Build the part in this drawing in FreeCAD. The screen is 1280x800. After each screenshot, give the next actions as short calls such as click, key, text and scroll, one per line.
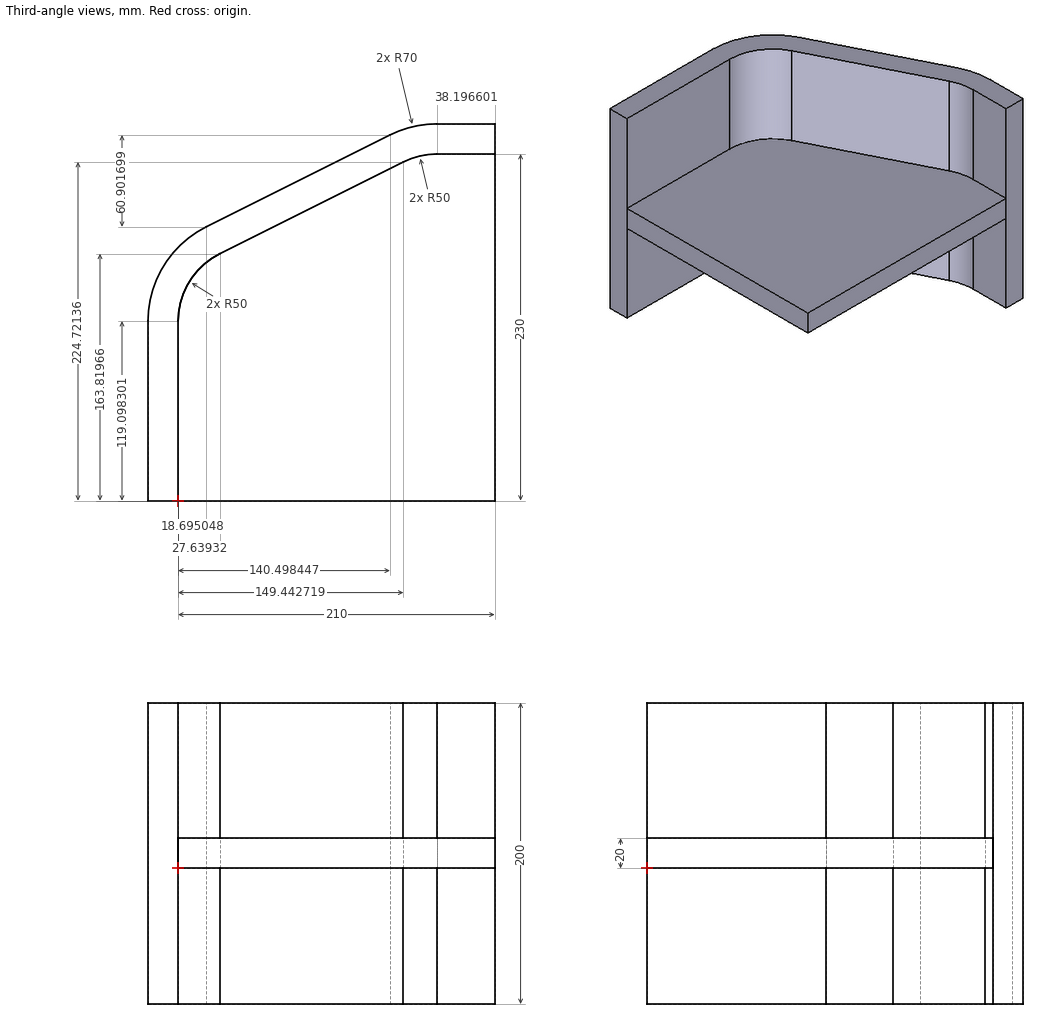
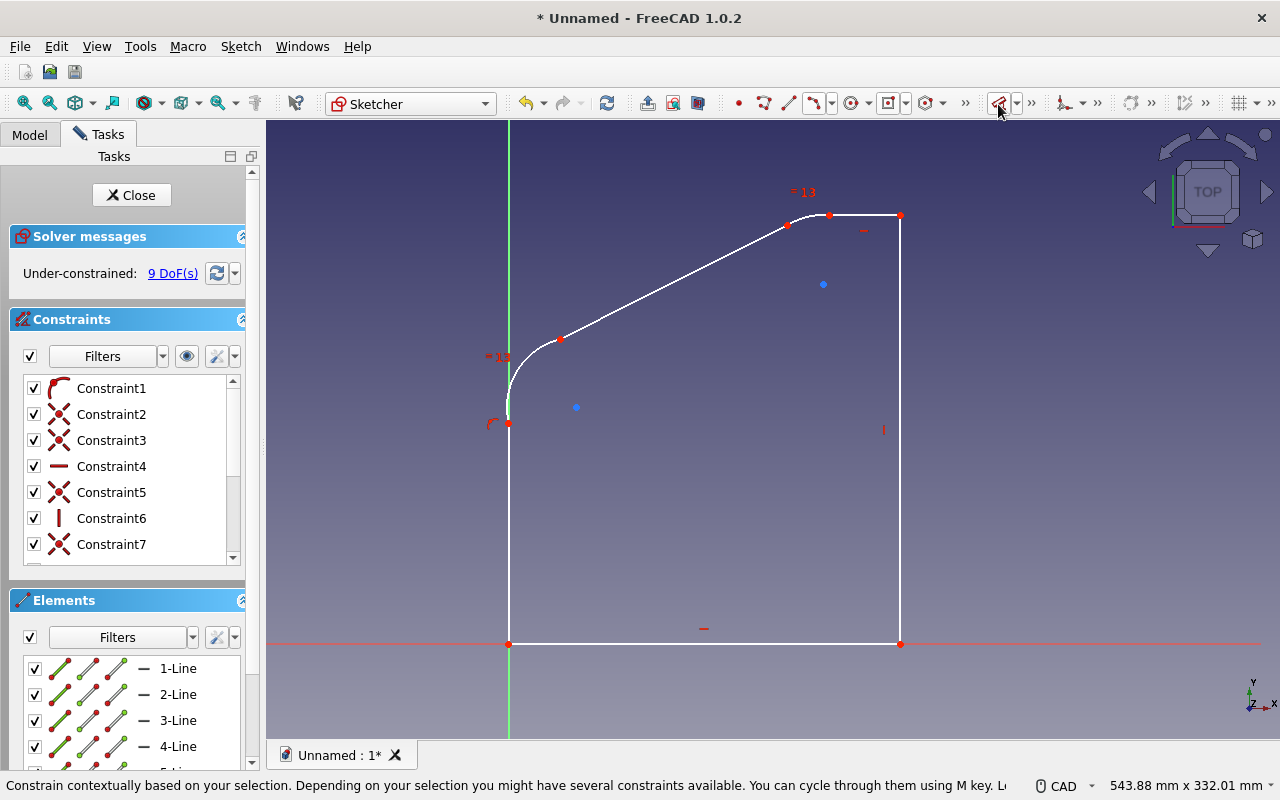
click(531, 354)
click(555, 307)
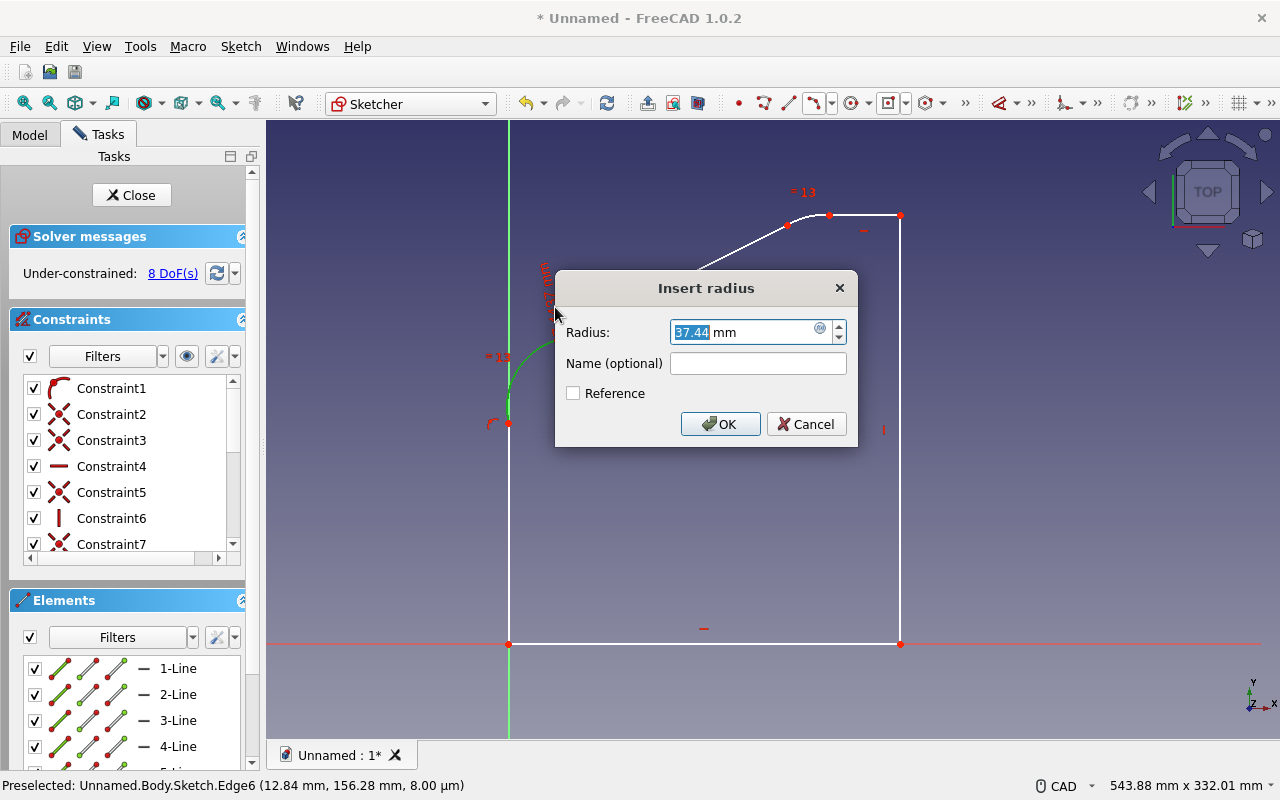
text(50)
key(Return)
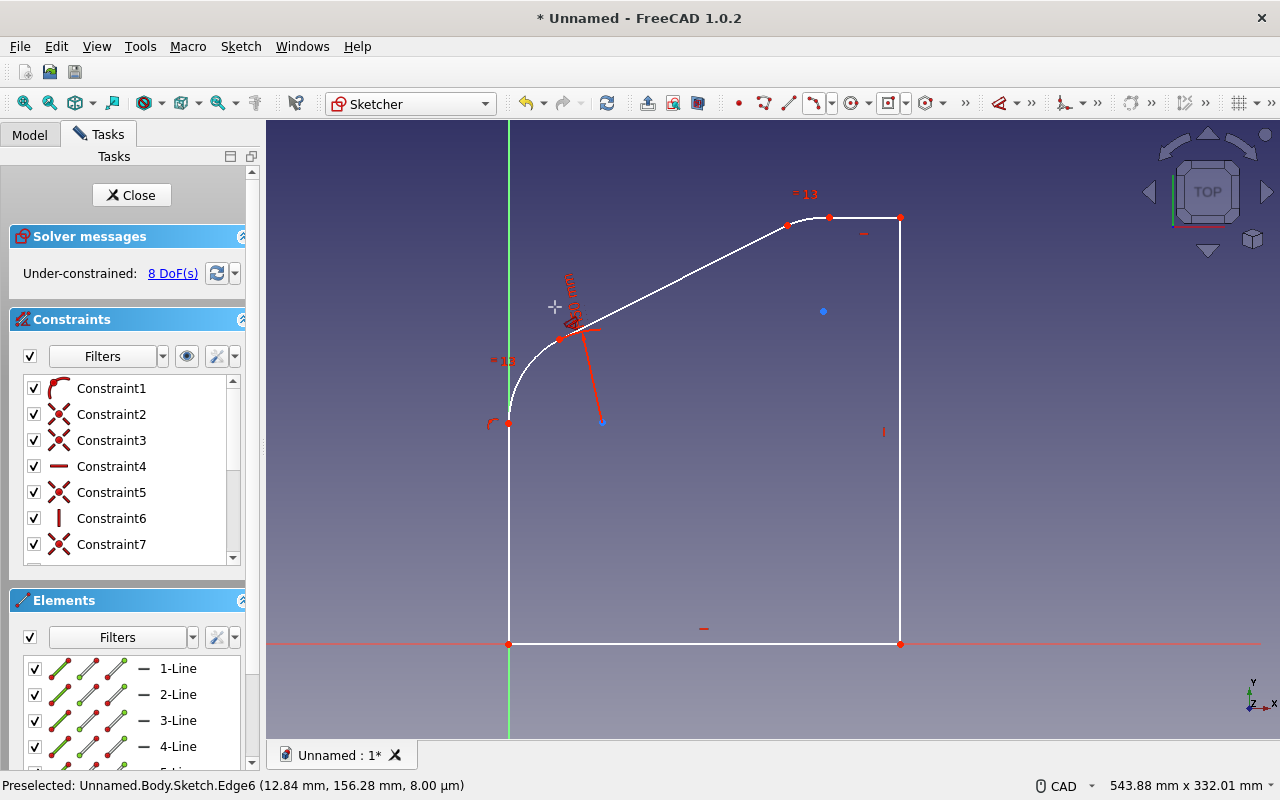
click(626, 644)
click(704, 678)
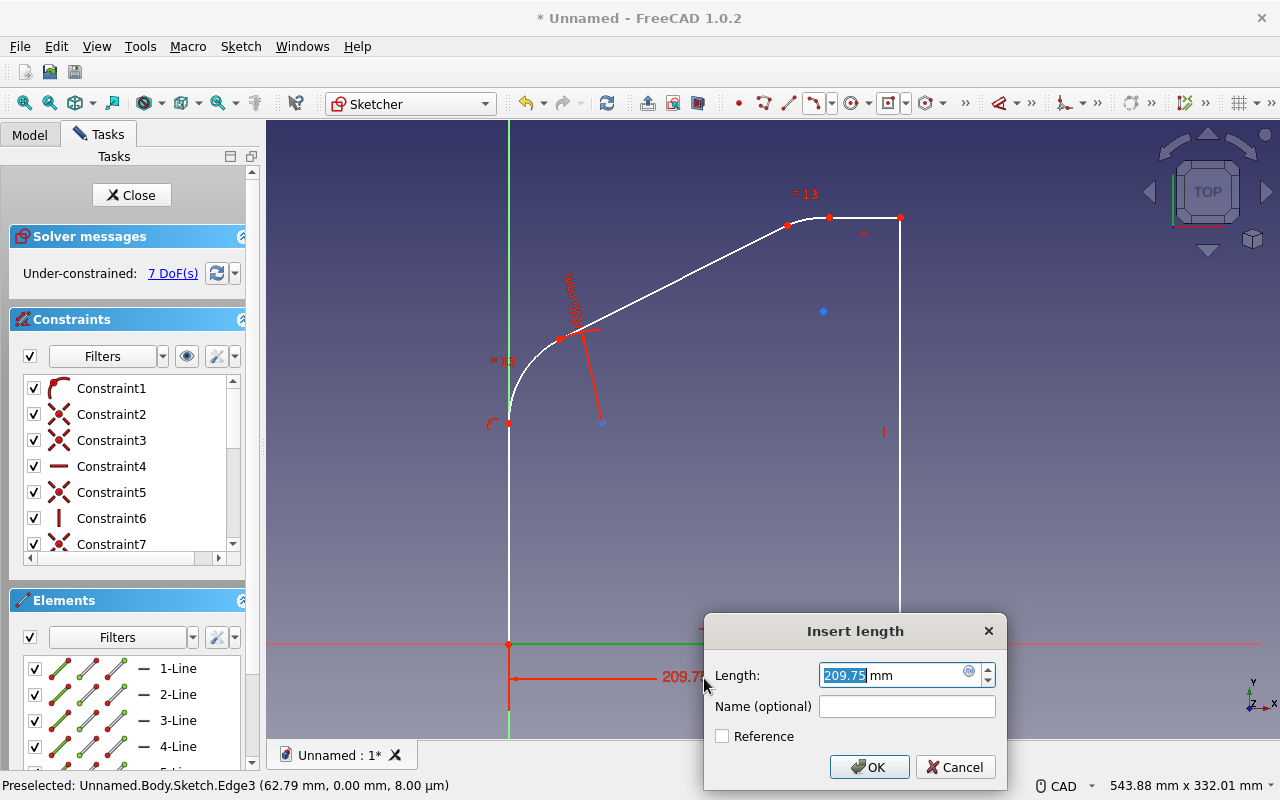
text(210)
key(Return)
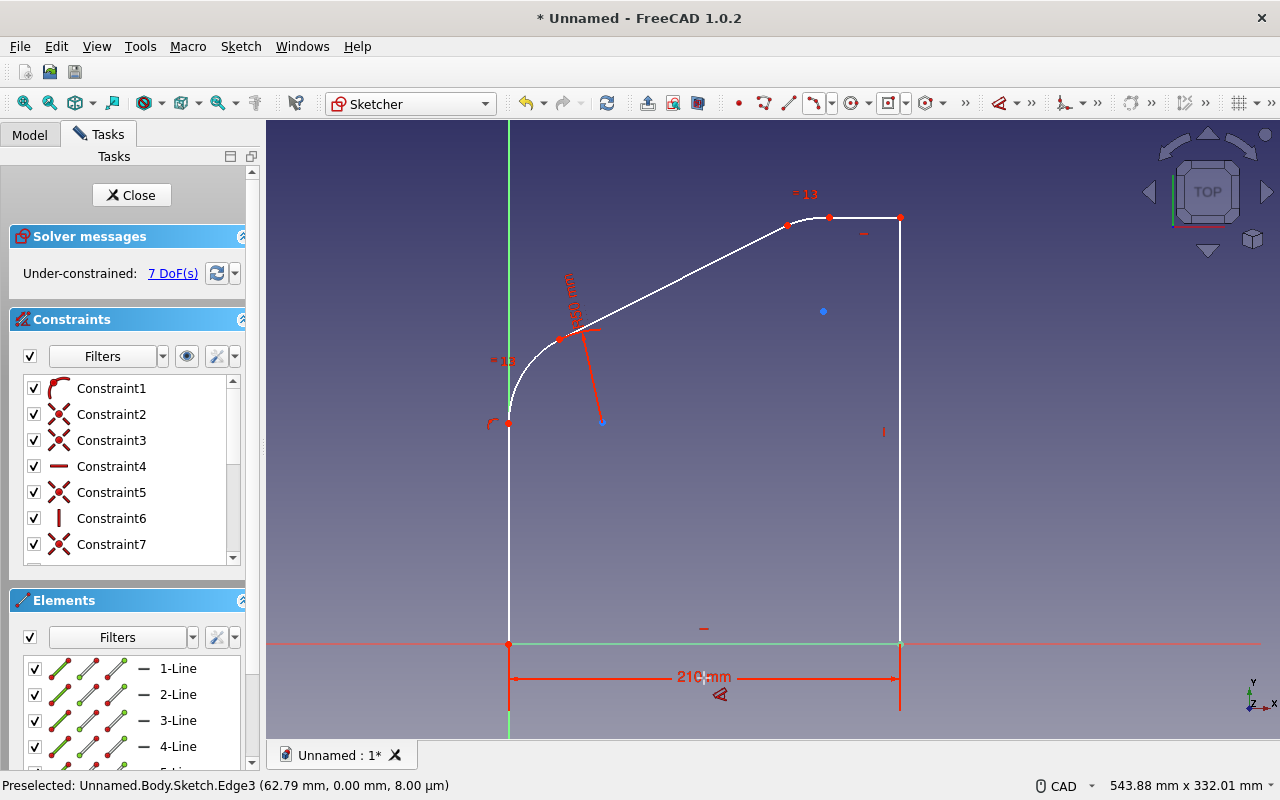
click(900, 516)
click(934, 431)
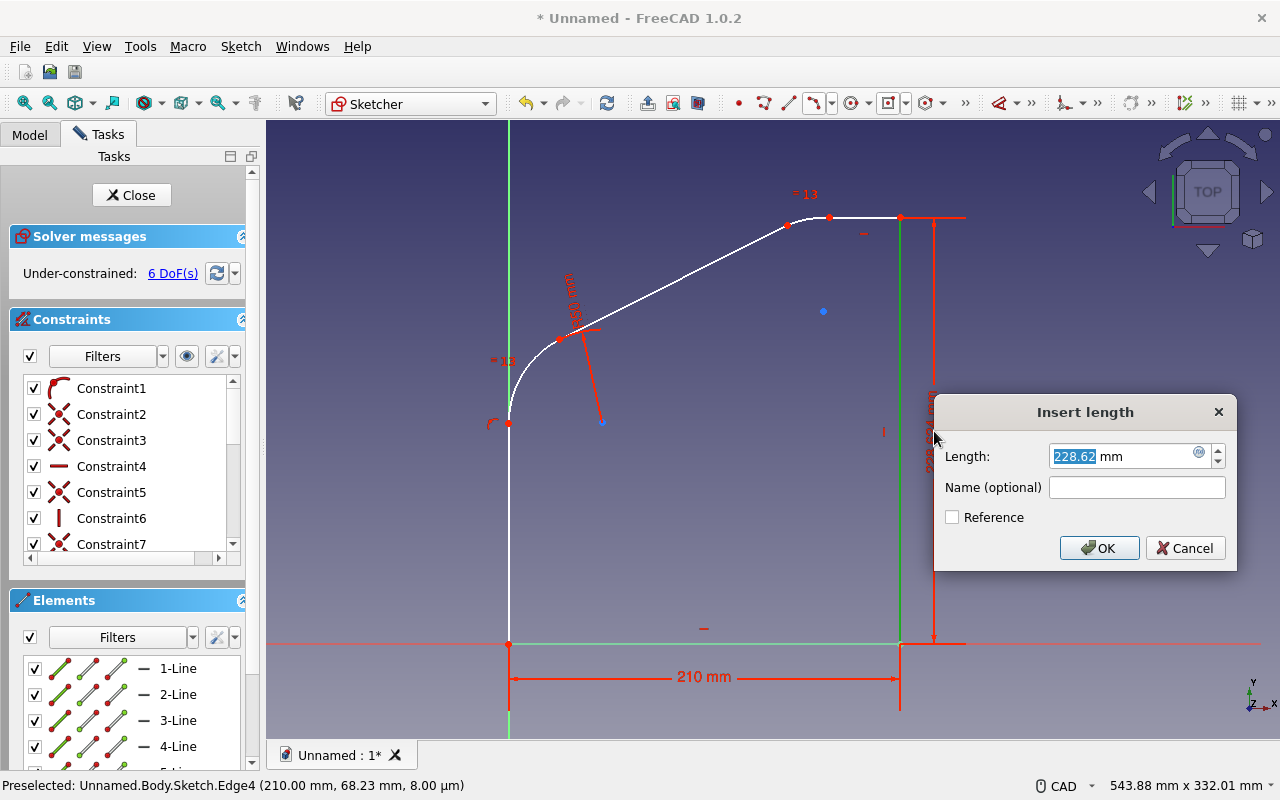
text(230)
key(Return)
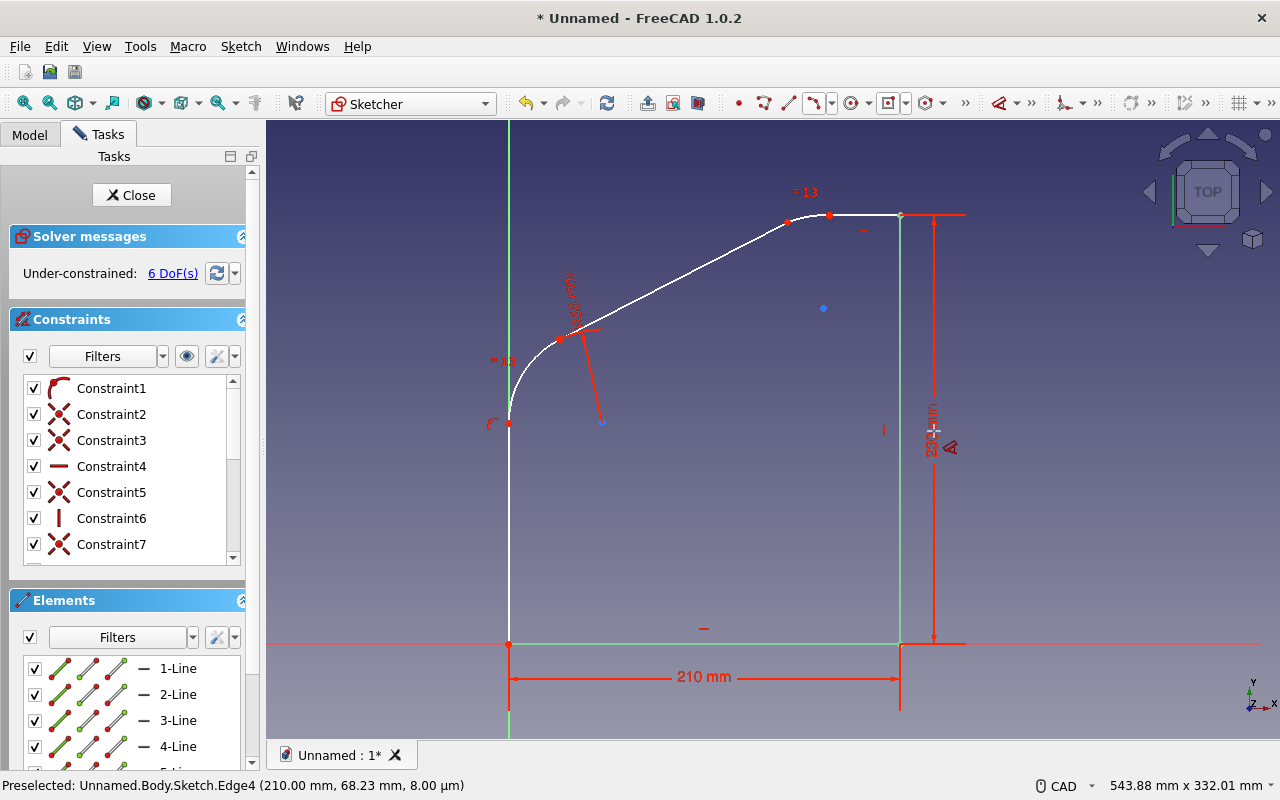
click(879, 215)
click(865, 181)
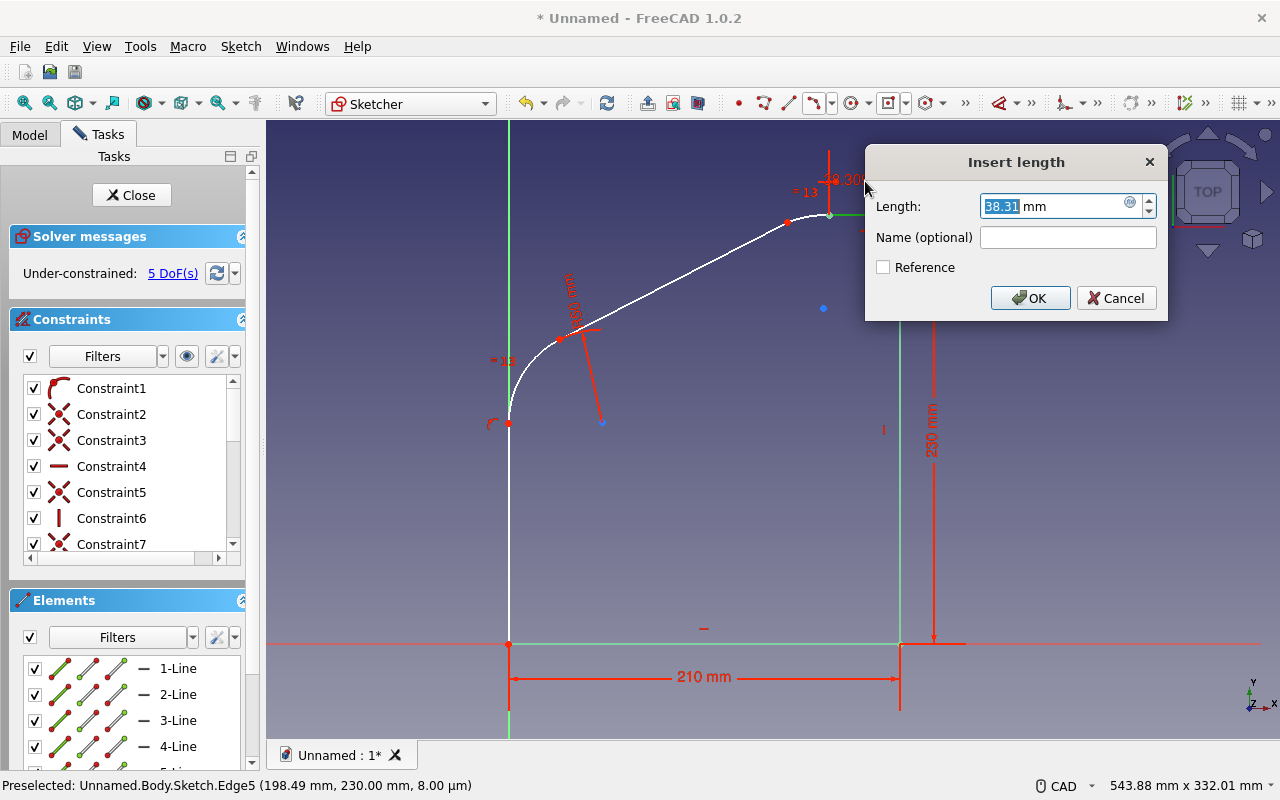
text(38.196601)
key(Return)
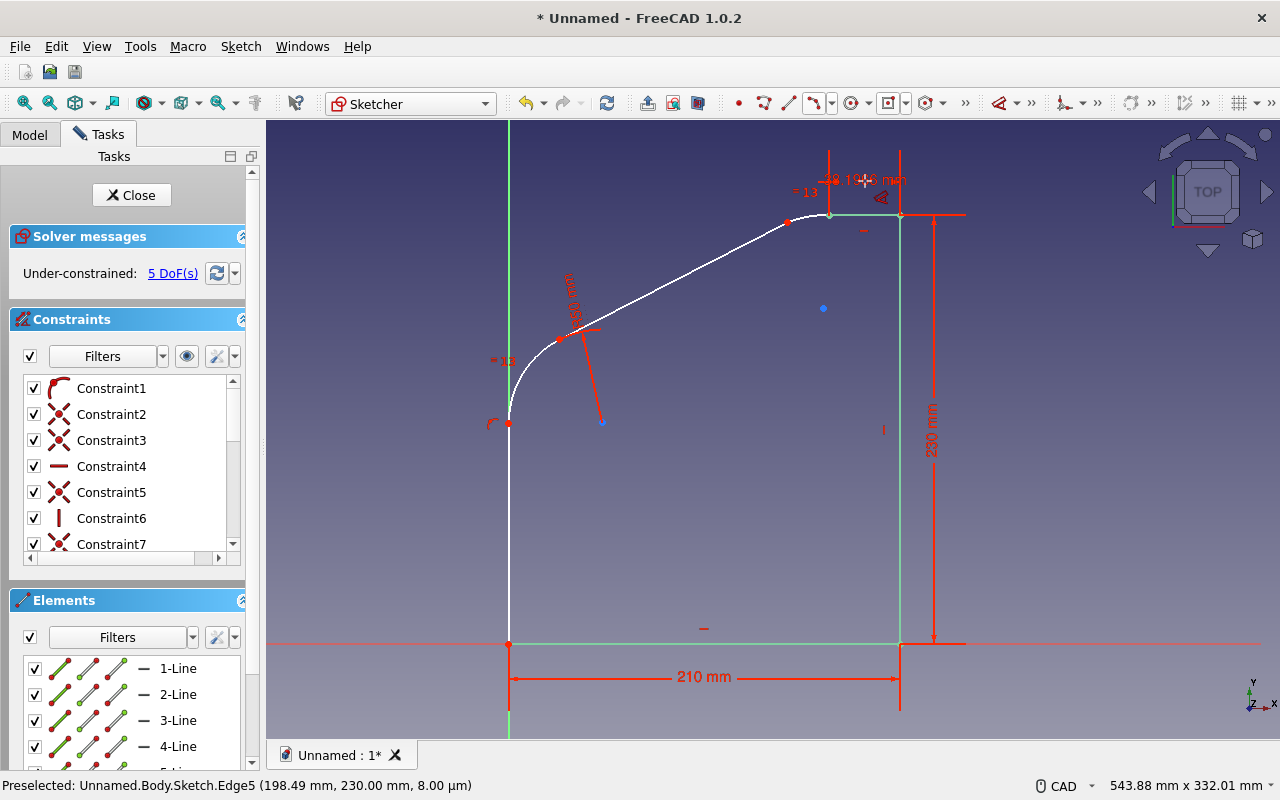
click(560, 340)
click(534, 678)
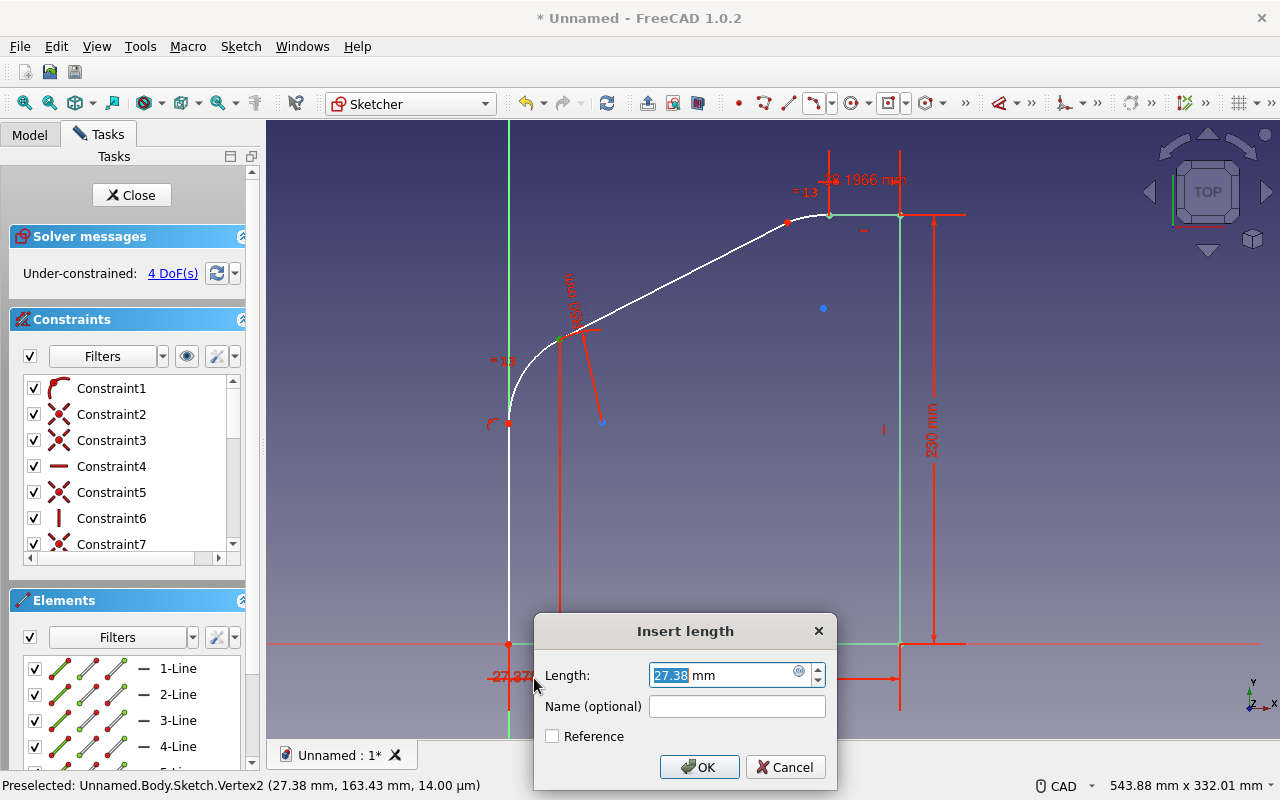
text(27.63932)
key(Return)